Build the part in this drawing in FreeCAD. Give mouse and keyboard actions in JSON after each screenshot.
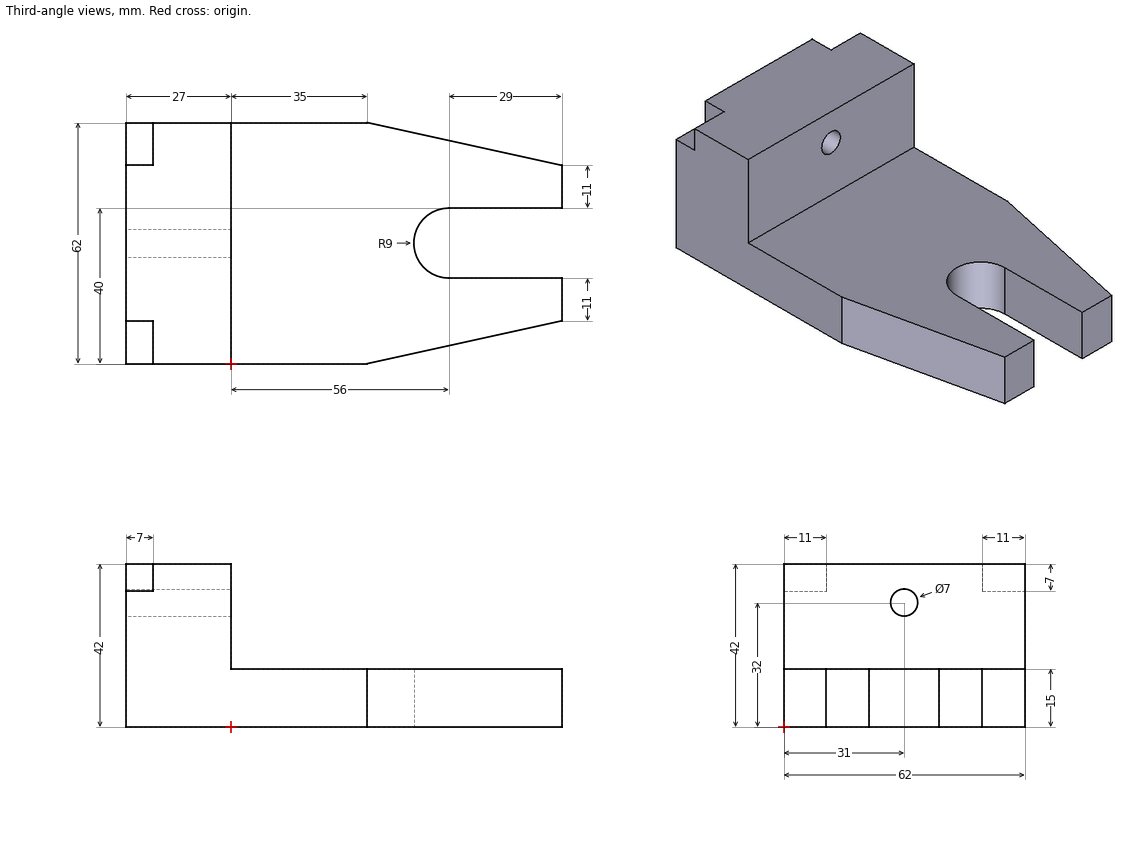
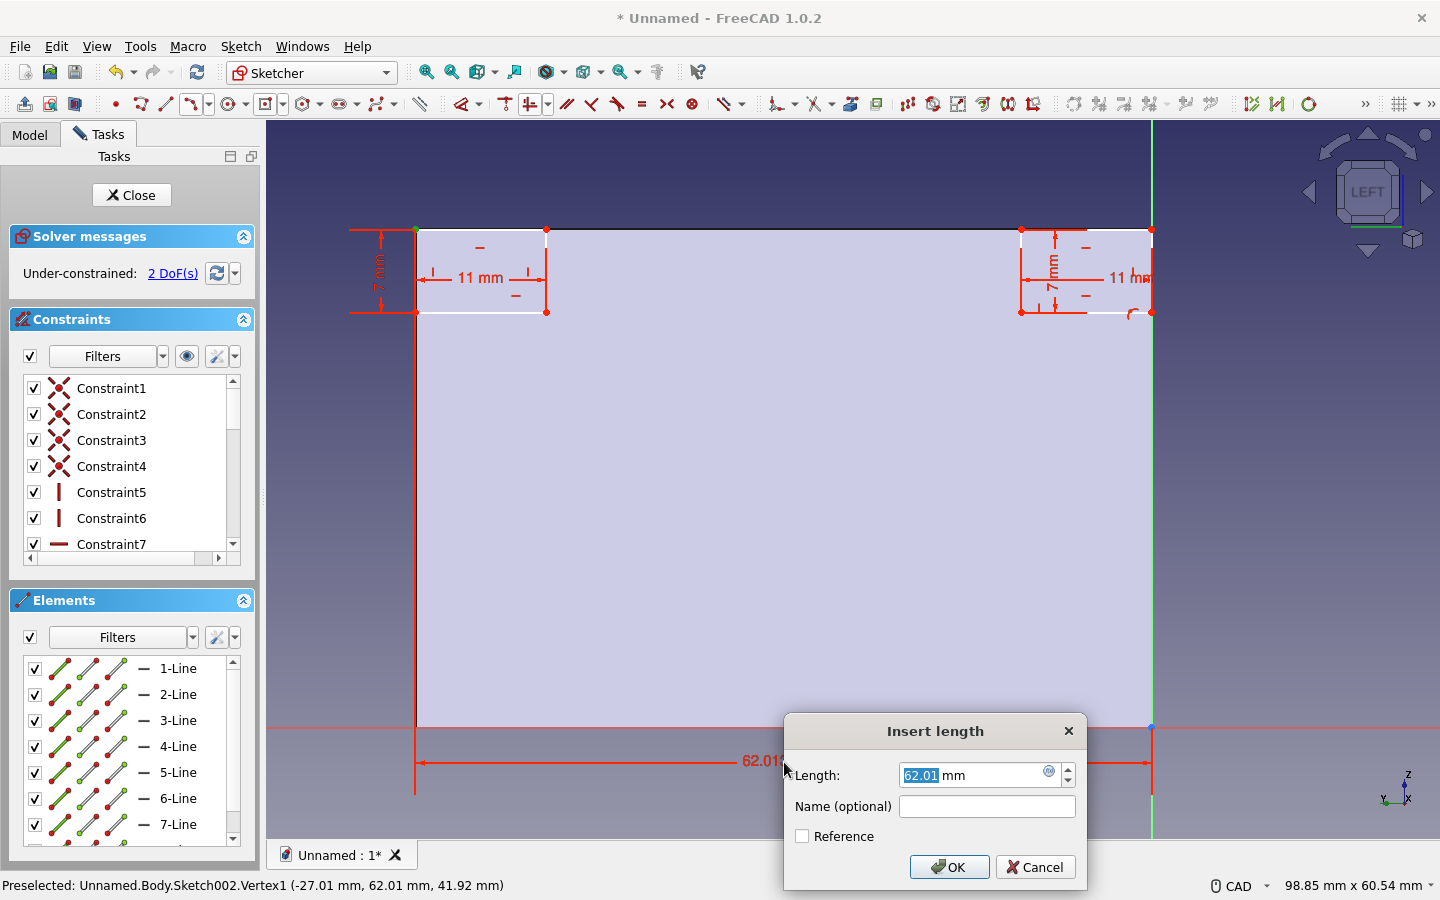
{"action": "type", "text": "62"}
{"action": "key", "text": "Return"}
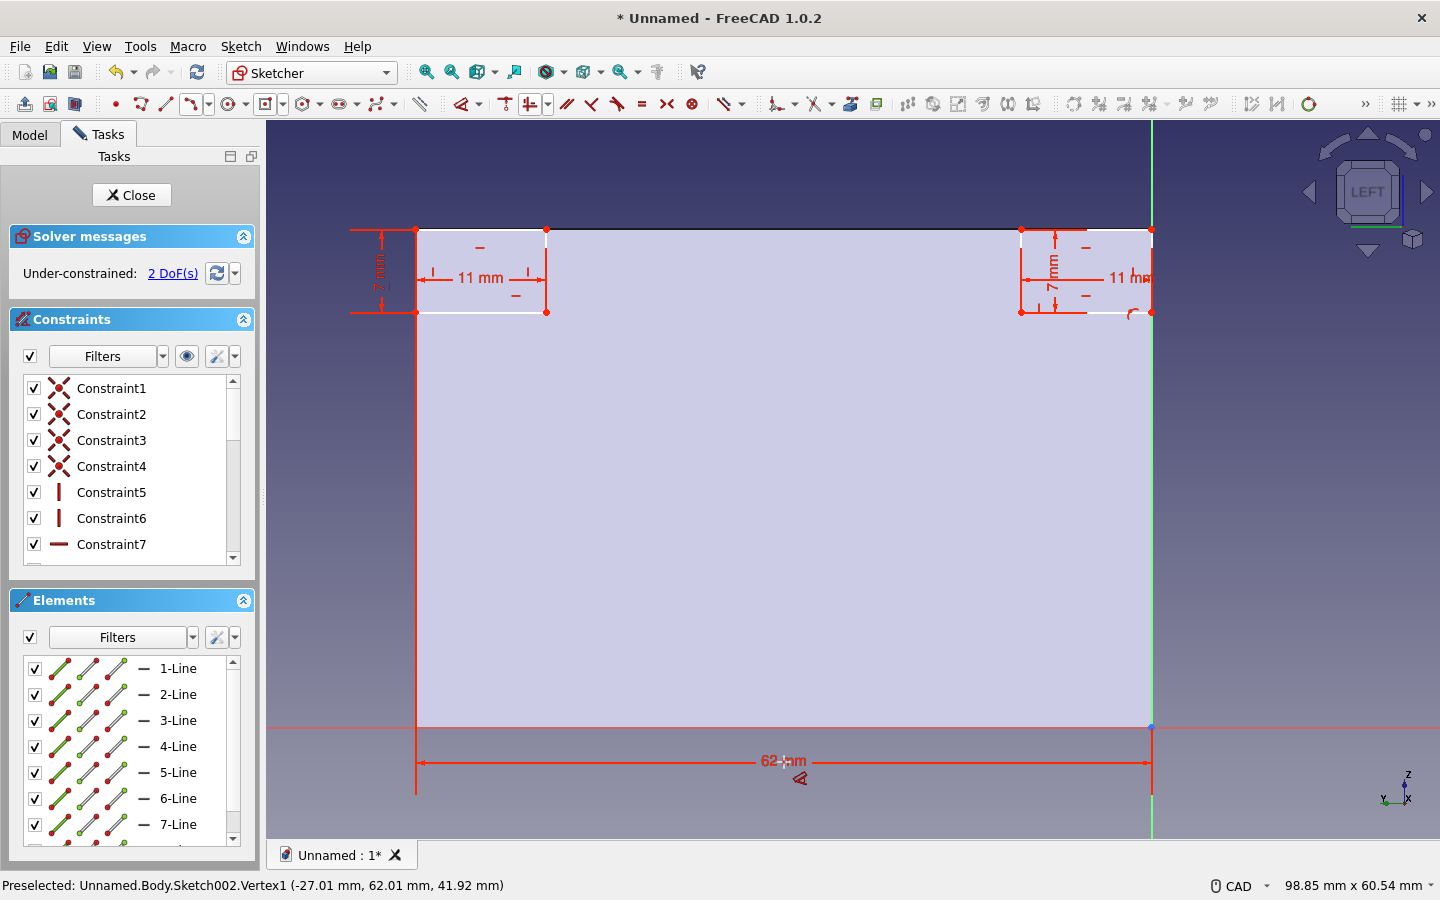
{"action": "left_click", "coordinate": [416, 230]}
{"action": "left_click", "coordinate": [1186, 479]}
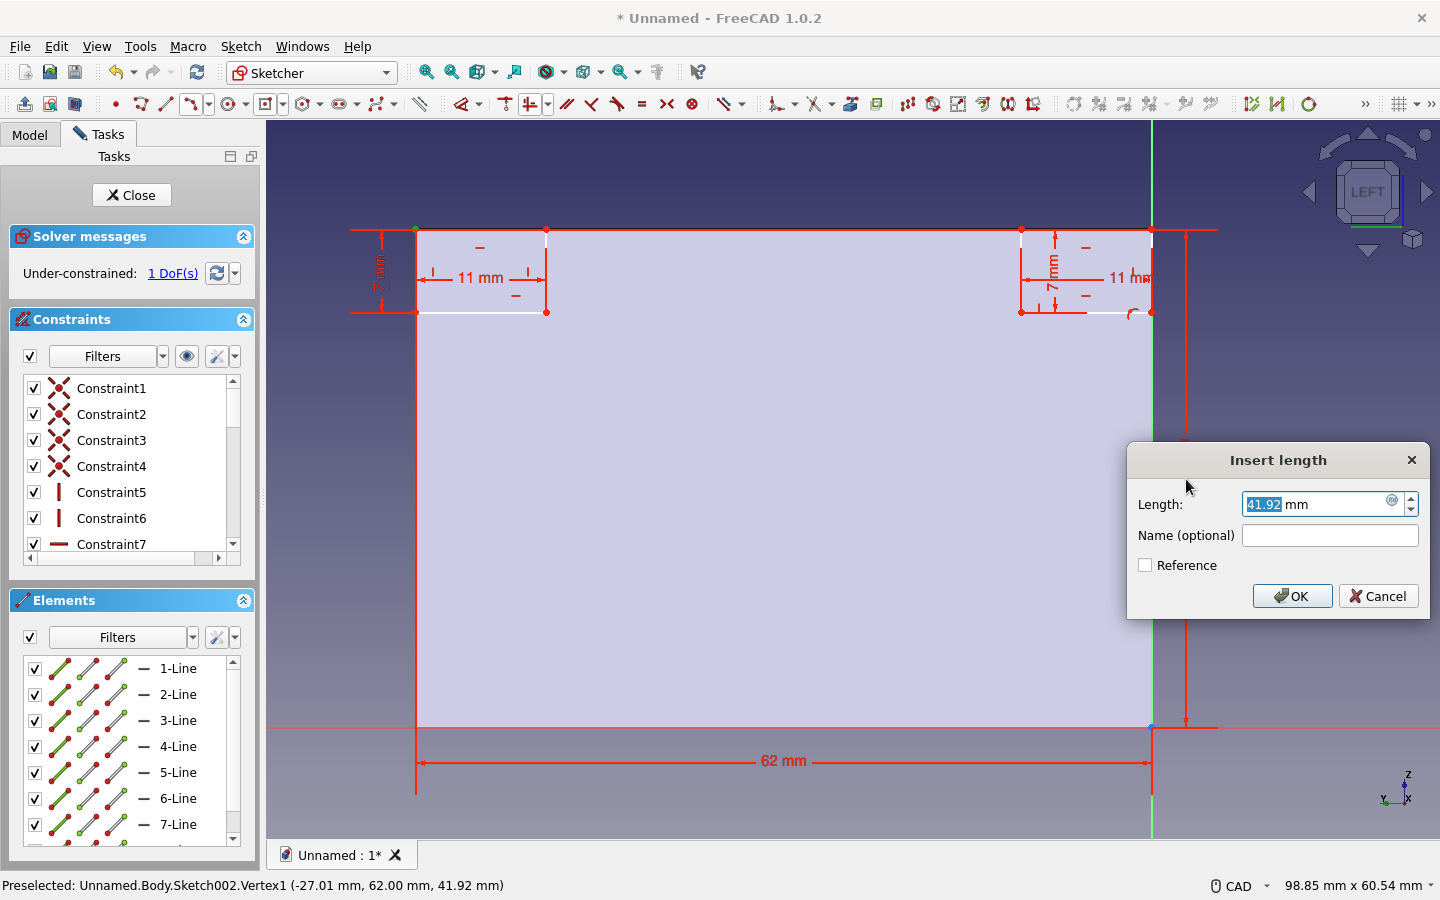
{"action": "type", "text": "42"}
{"action": "key", "text": "Return"}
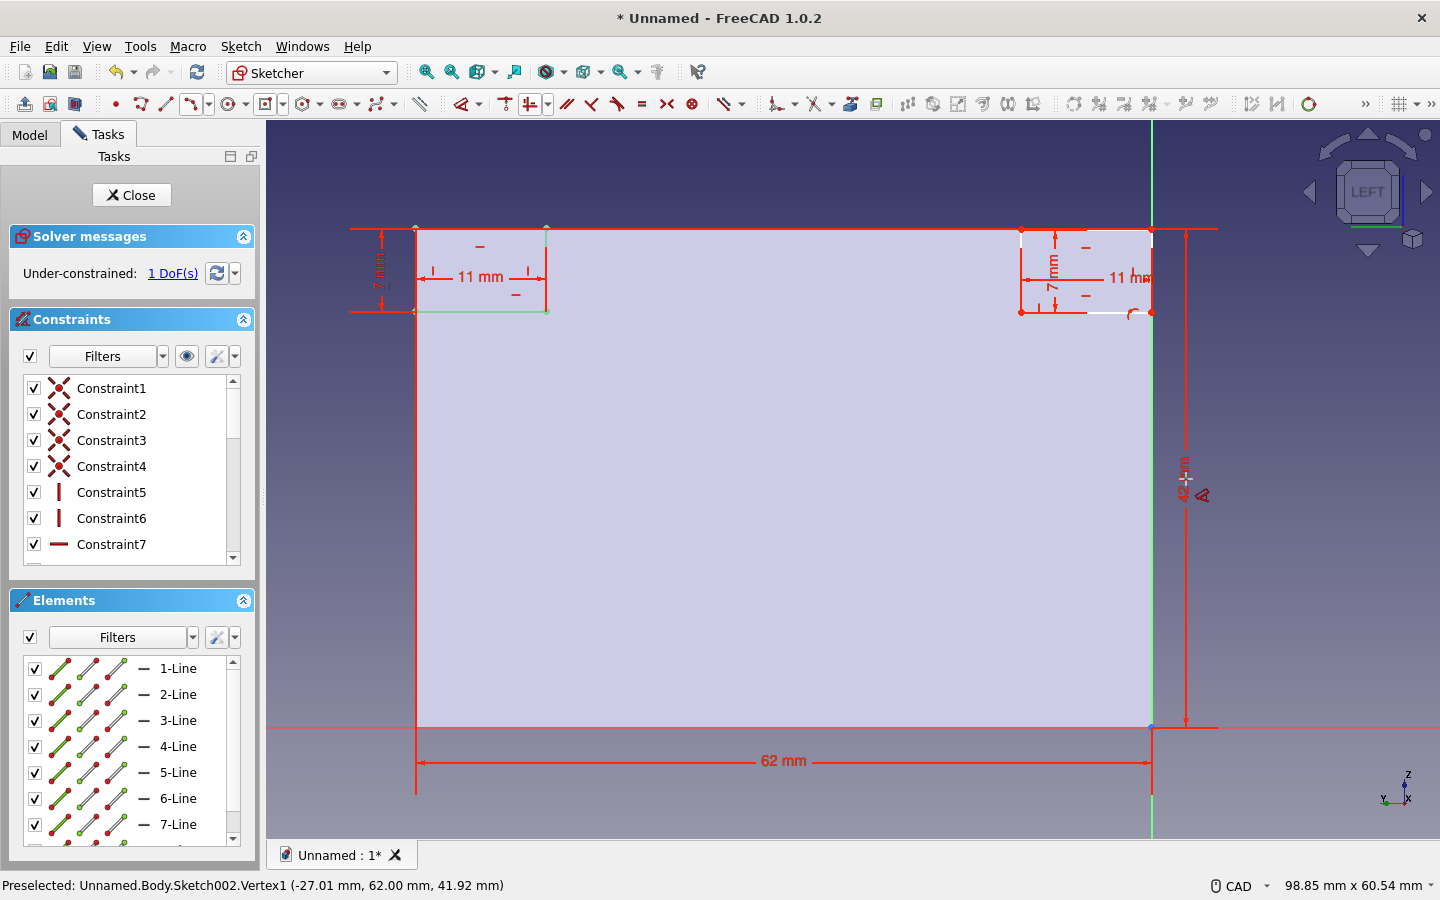
{"action": "left_click", "coordinate": [1021, 230]}
{"action": "left_click", "coordinate": [1186, 364]}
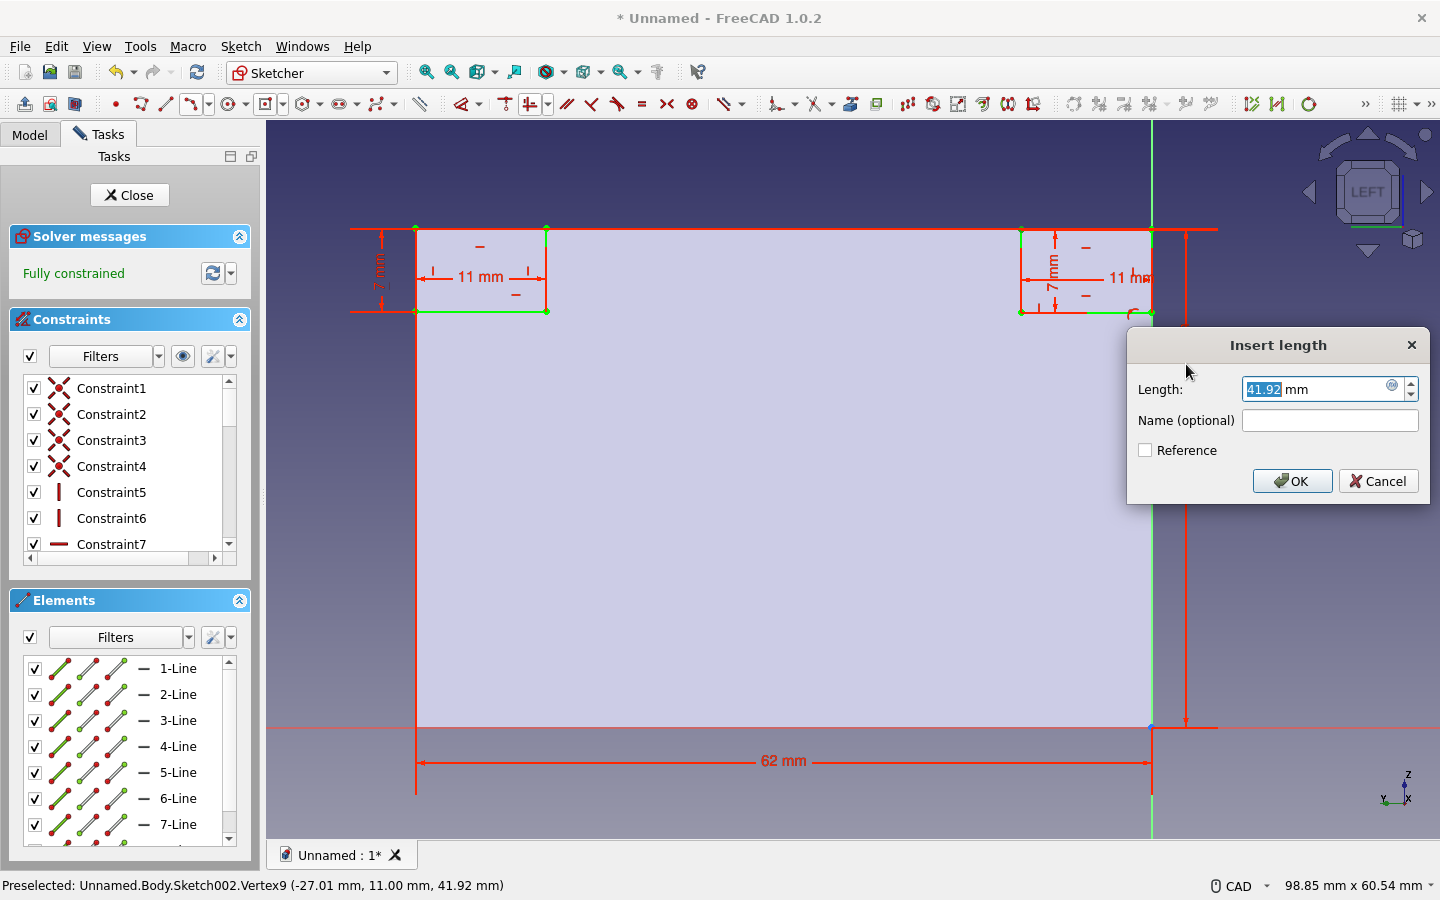
{"action": "type", "text": "42"}
{"action": "key", "text": "Return"}
{"action": "key", "text": "Escape"}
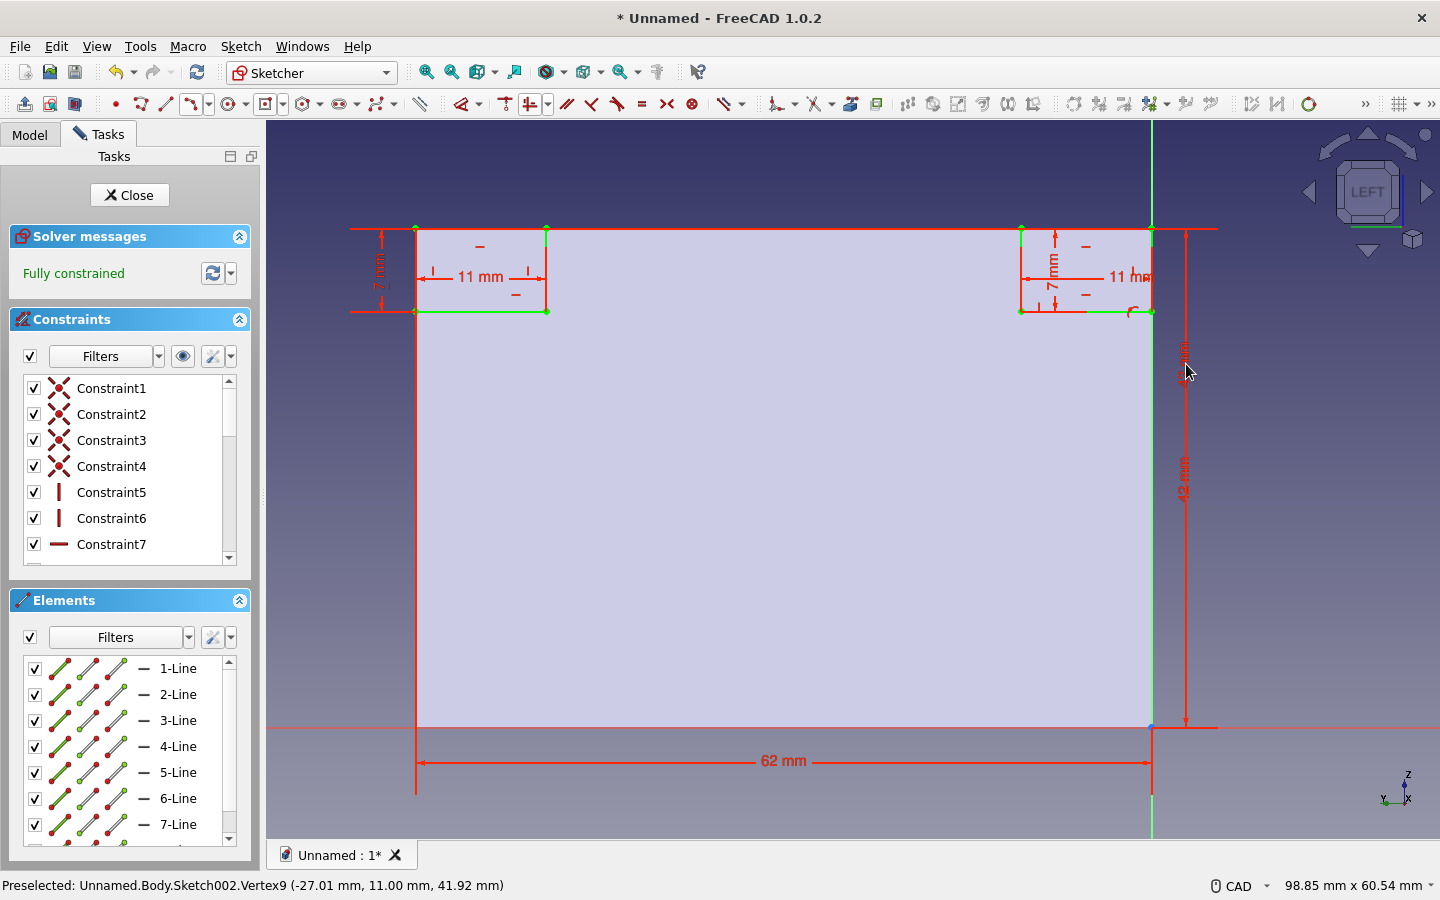
{"action": "left_click", "coordinate": [130, 195]}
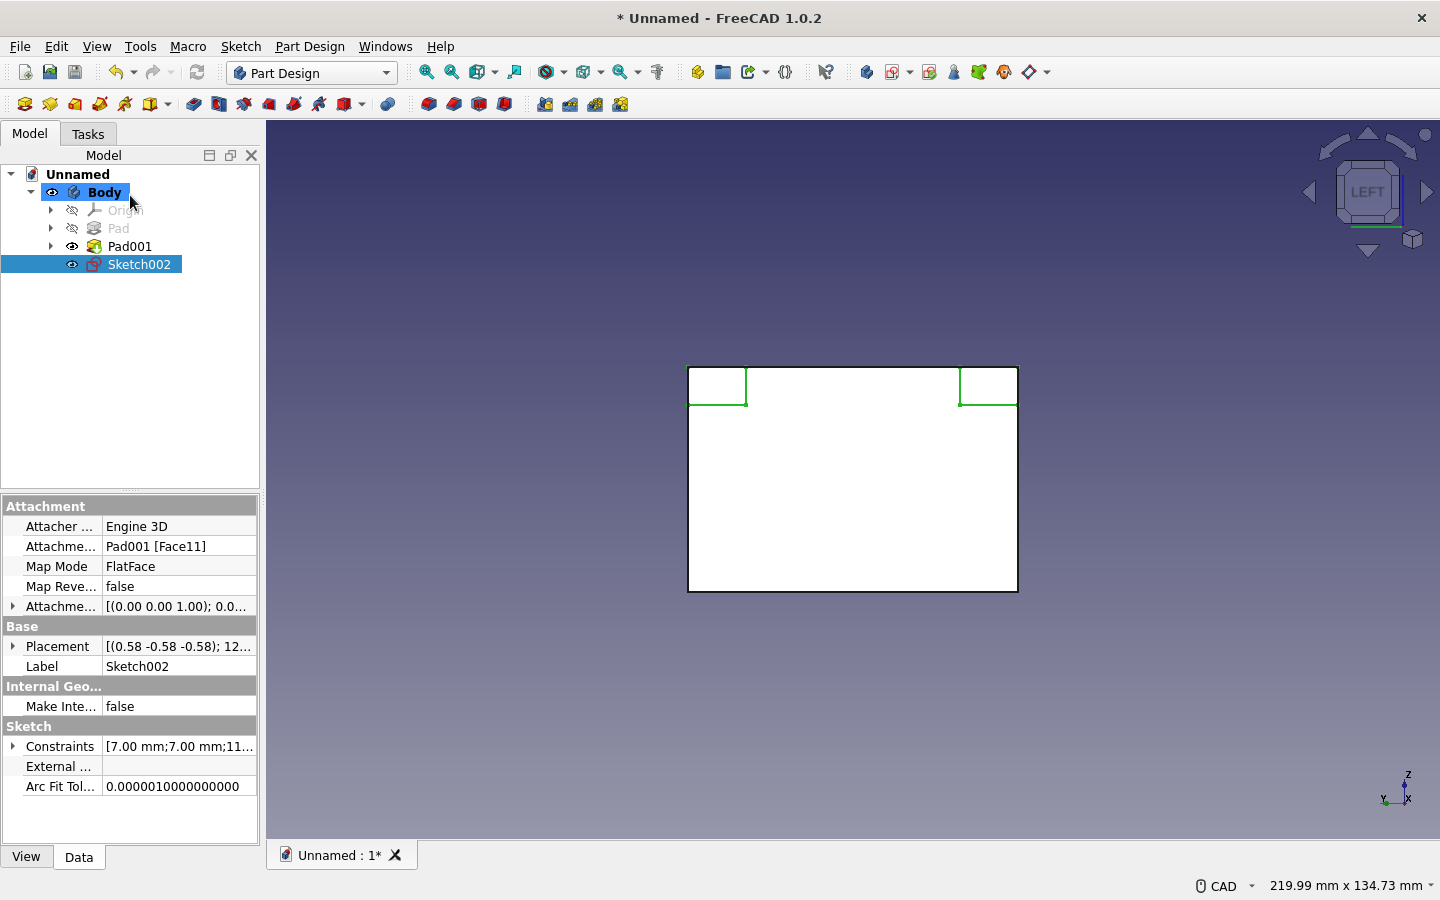
{"action": "left_click", "coordinate": [194, 104]}